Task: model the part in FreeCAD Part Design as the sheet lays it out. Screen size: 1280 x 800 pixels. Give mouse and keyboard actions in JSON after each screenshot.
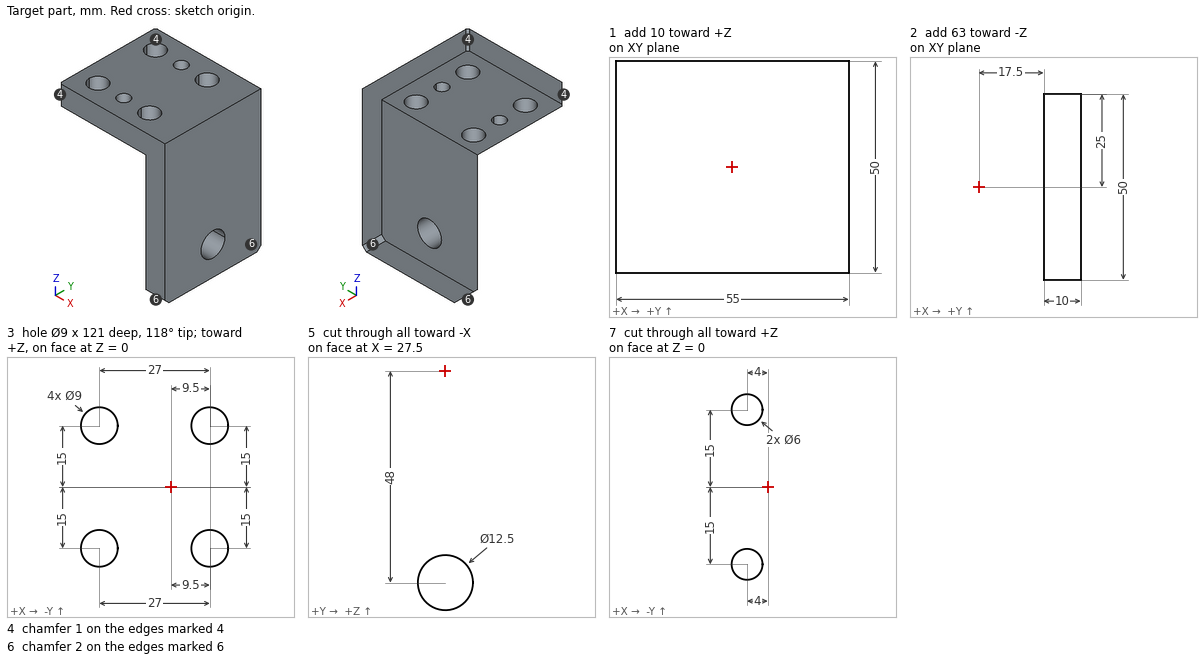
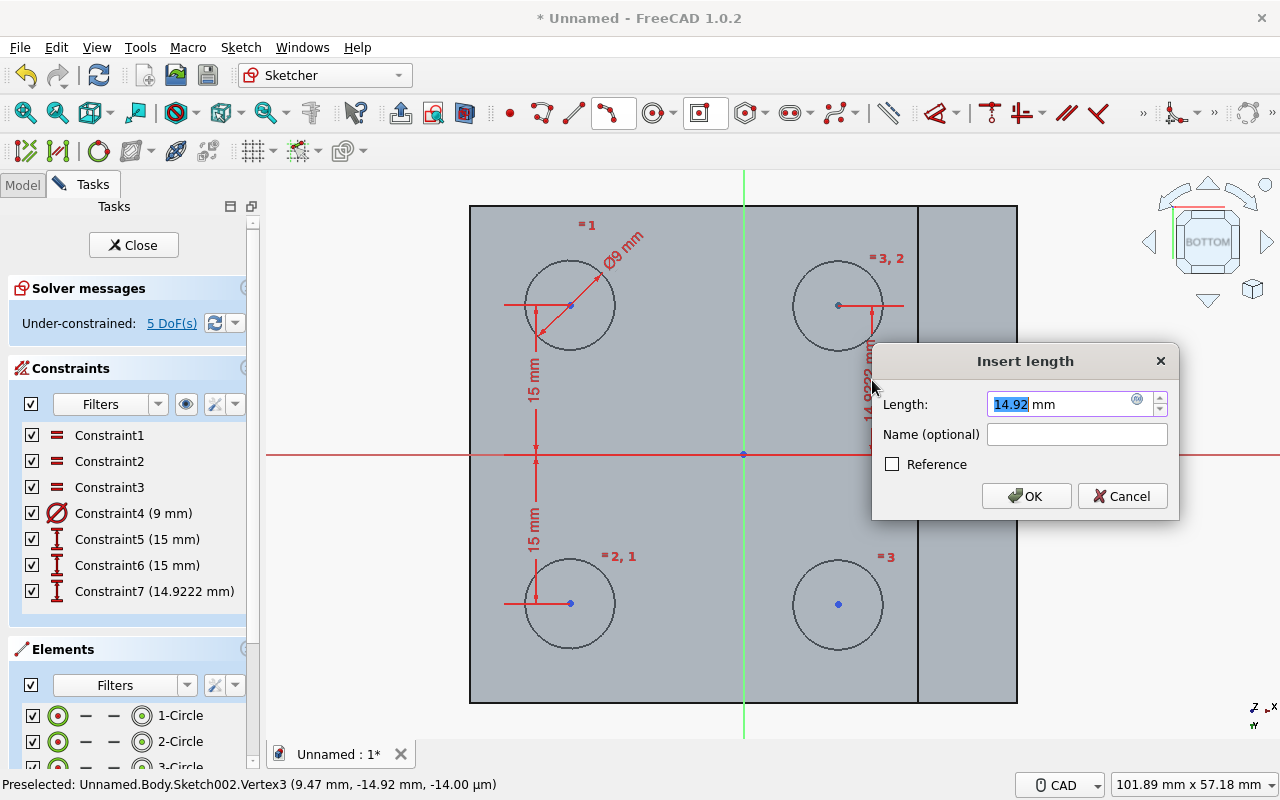
{"action": "type", "text": "15"}
{"action": "key", "text": "Return"}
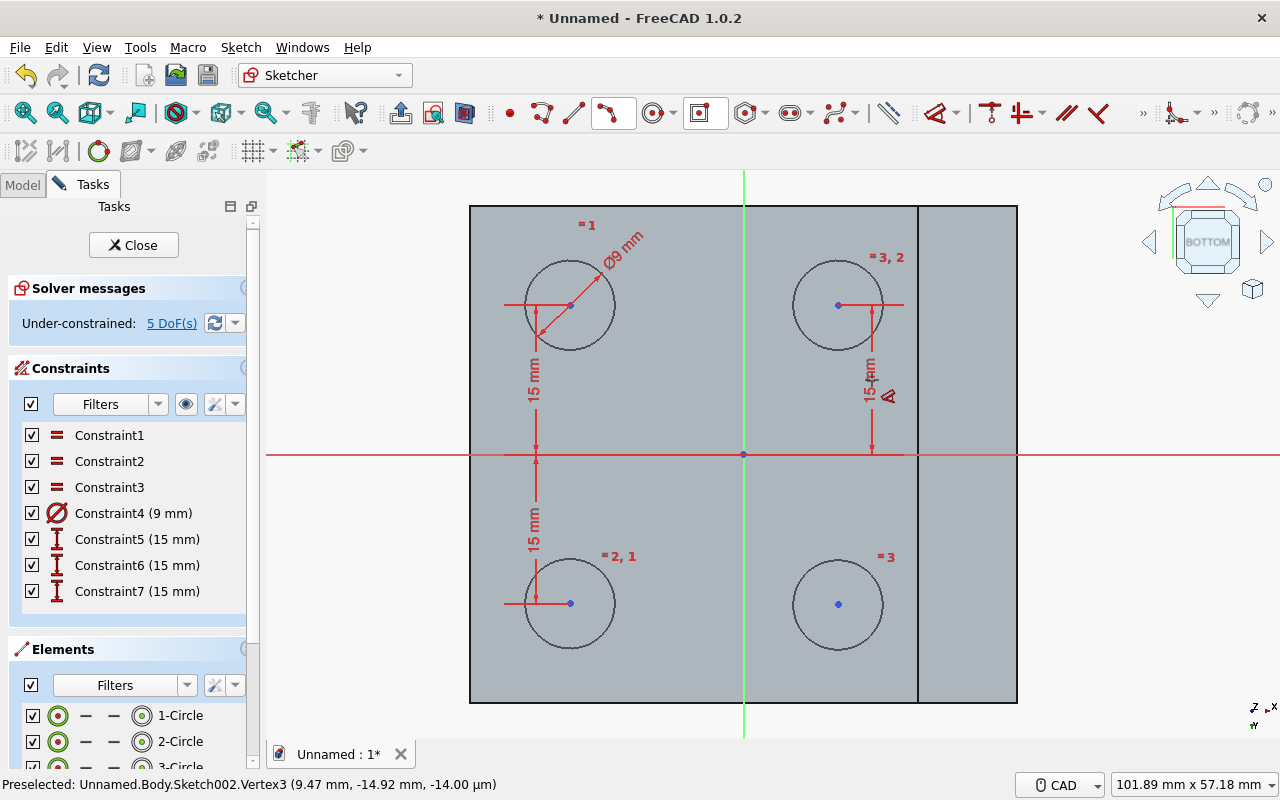
{"action": "left_click", "coordinate": [838, 605]}
{"action": "left_click", "coordinate": [872, 530]}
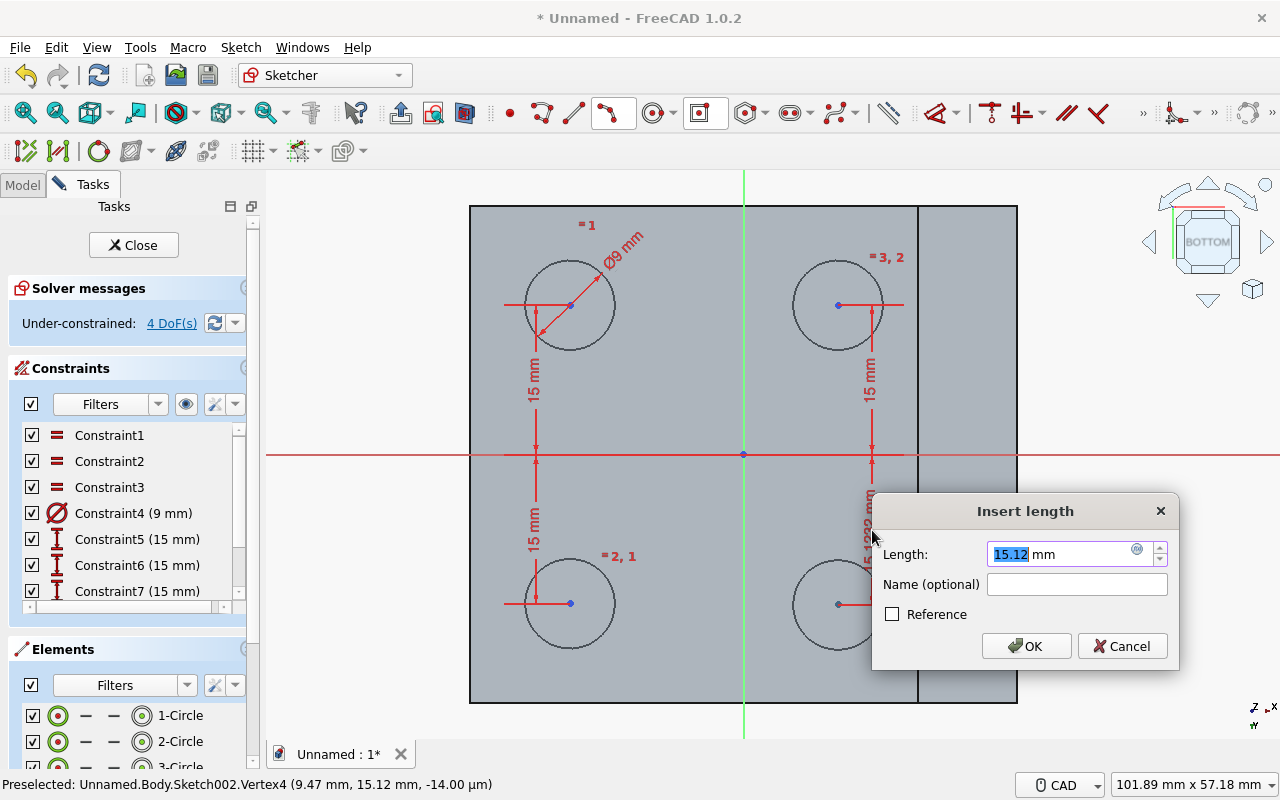
{"action": "type", "text": "15"}
{"action": "key", "text": "Return"}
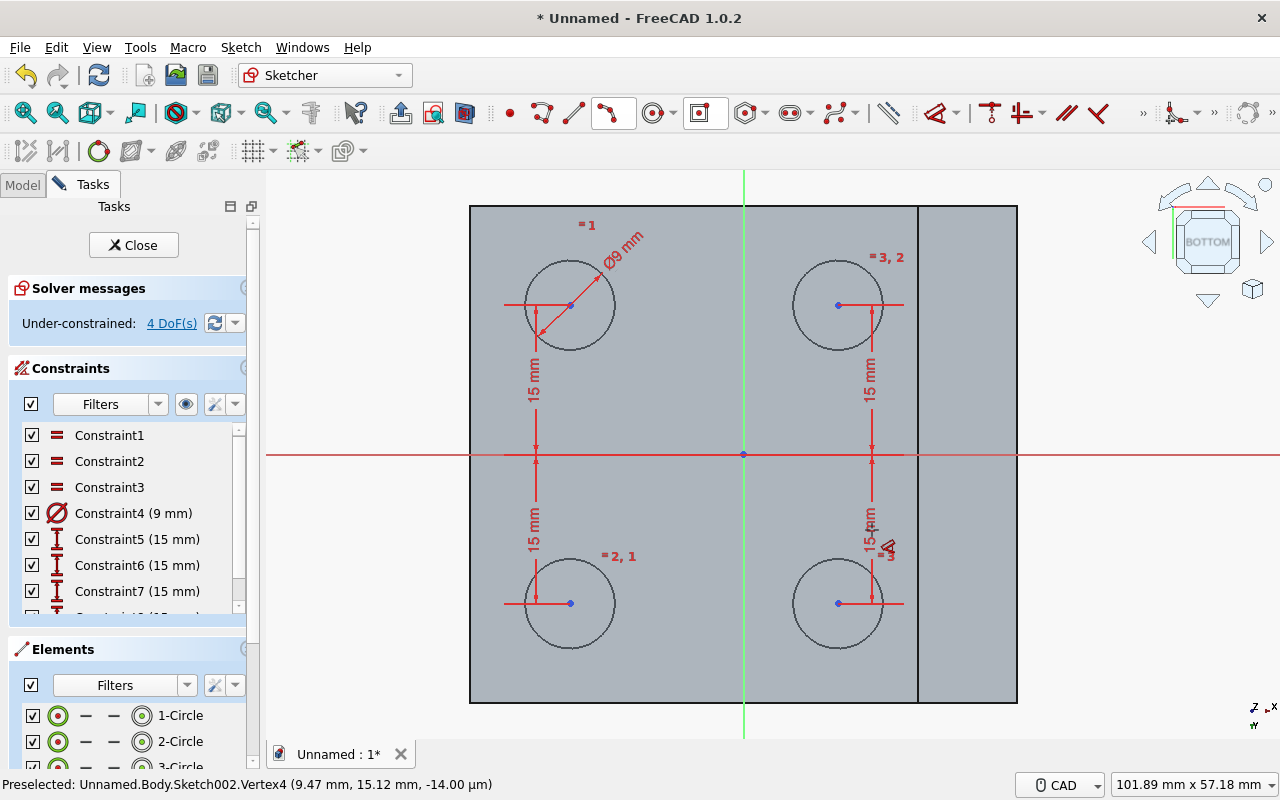
{"action": "left_click", "coordinate": [838, 305]}
{"action": "left_click", "coordinate": [791, 271]}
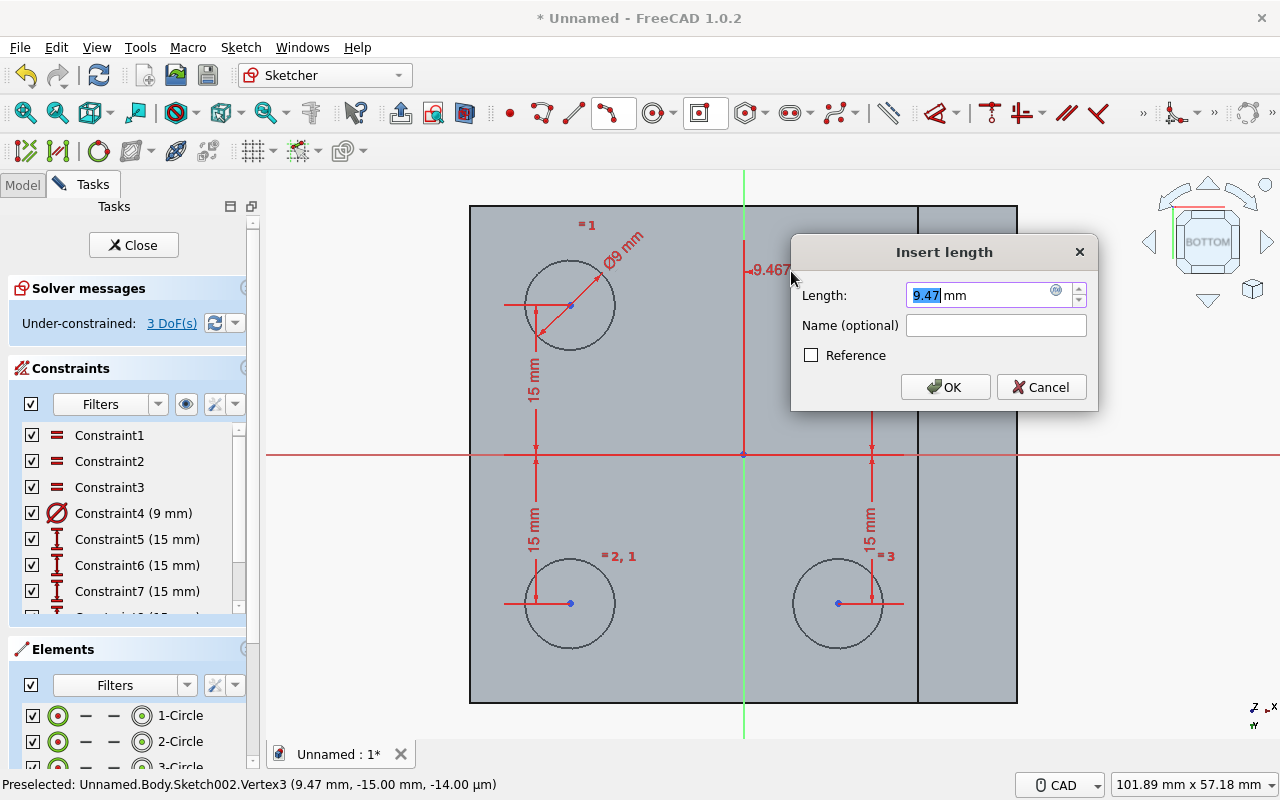
{"action": "type", "text": "9.5"}
{"action": "key", "text": "Return"}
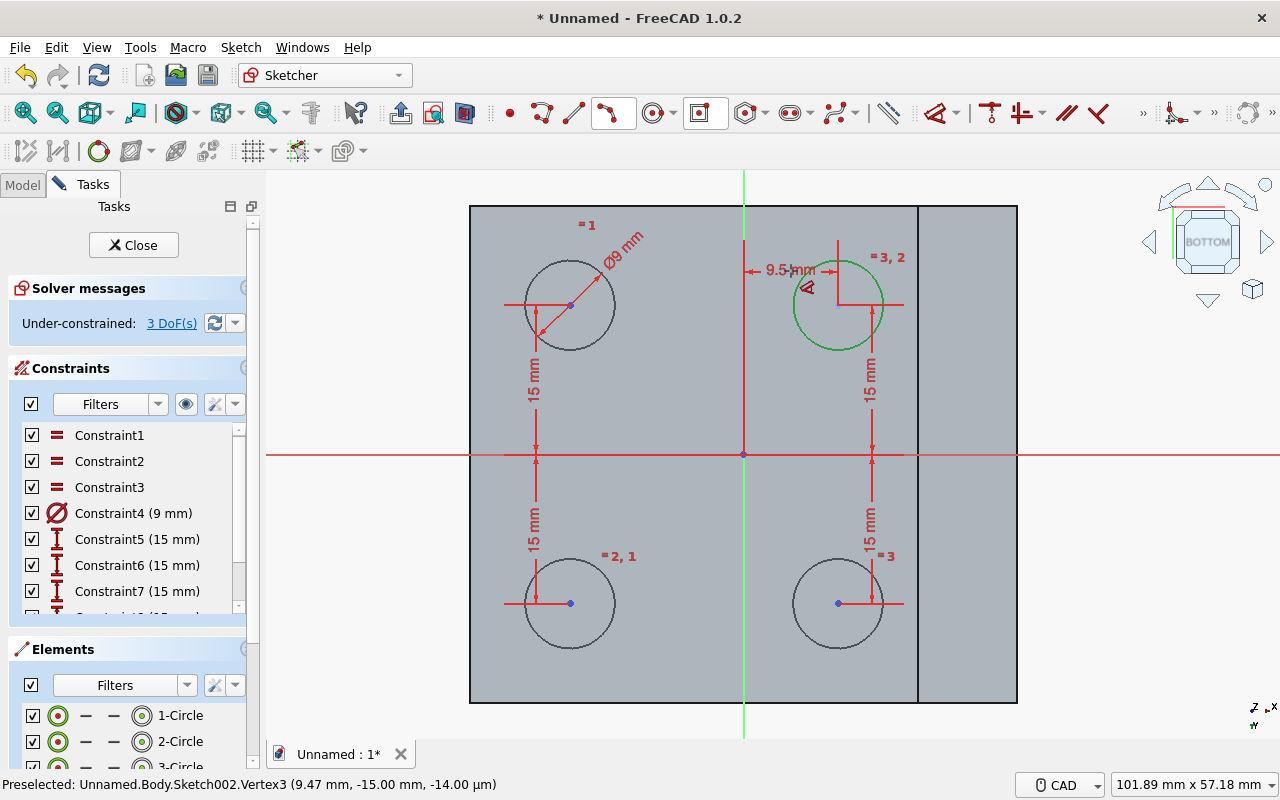
{"action": "left_click", "coordinate": [838, 604]}
{"action": "left_click", "coordinate": [791, 638]}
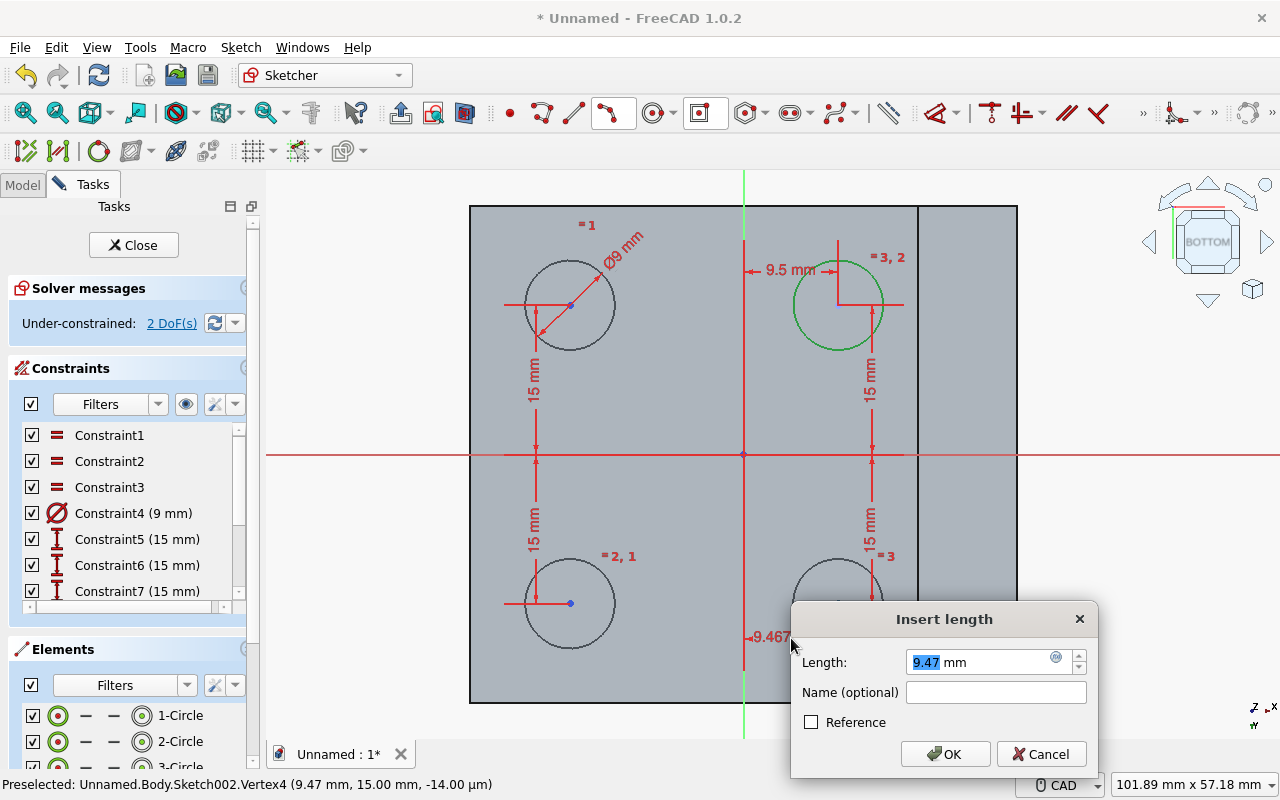
{"action": "type", "text": "9.5"}
{"action": "key", "text": "Return"}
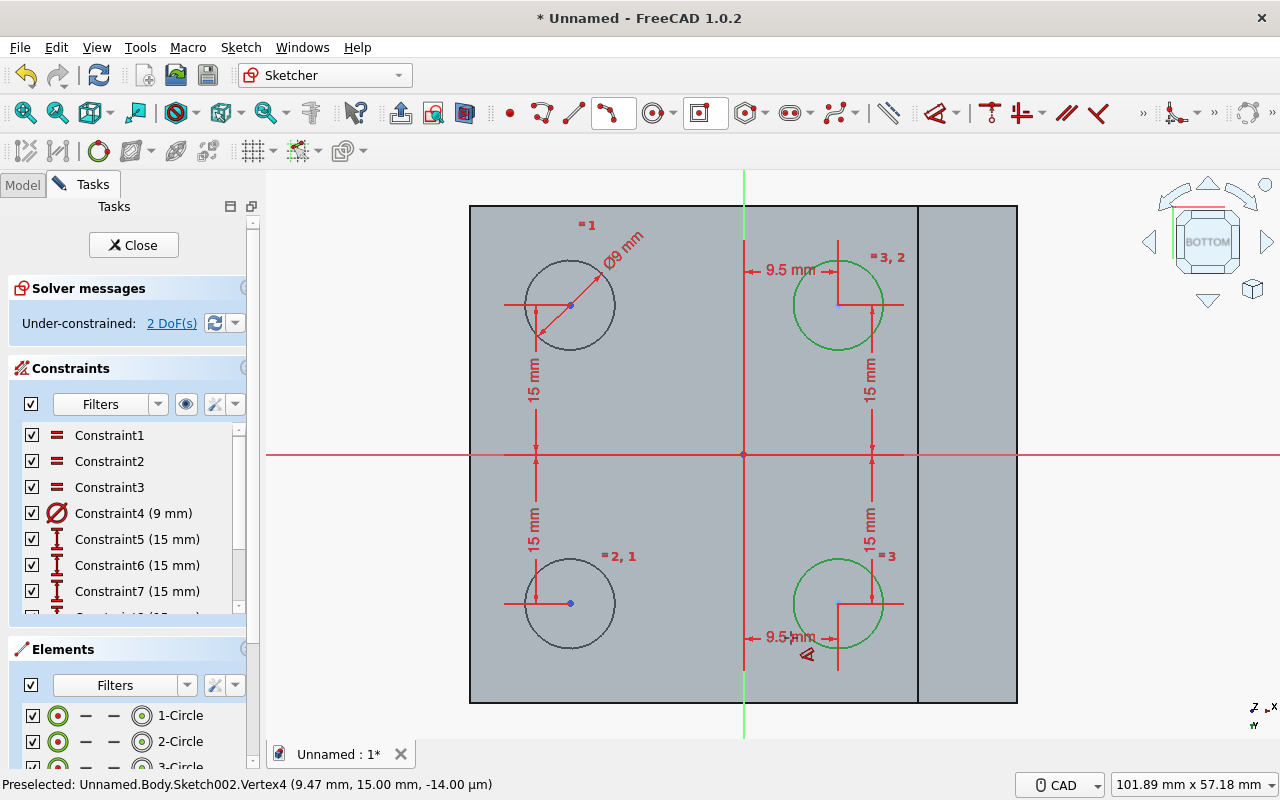
{"action": "left_click", "coordinate": [570, 305]}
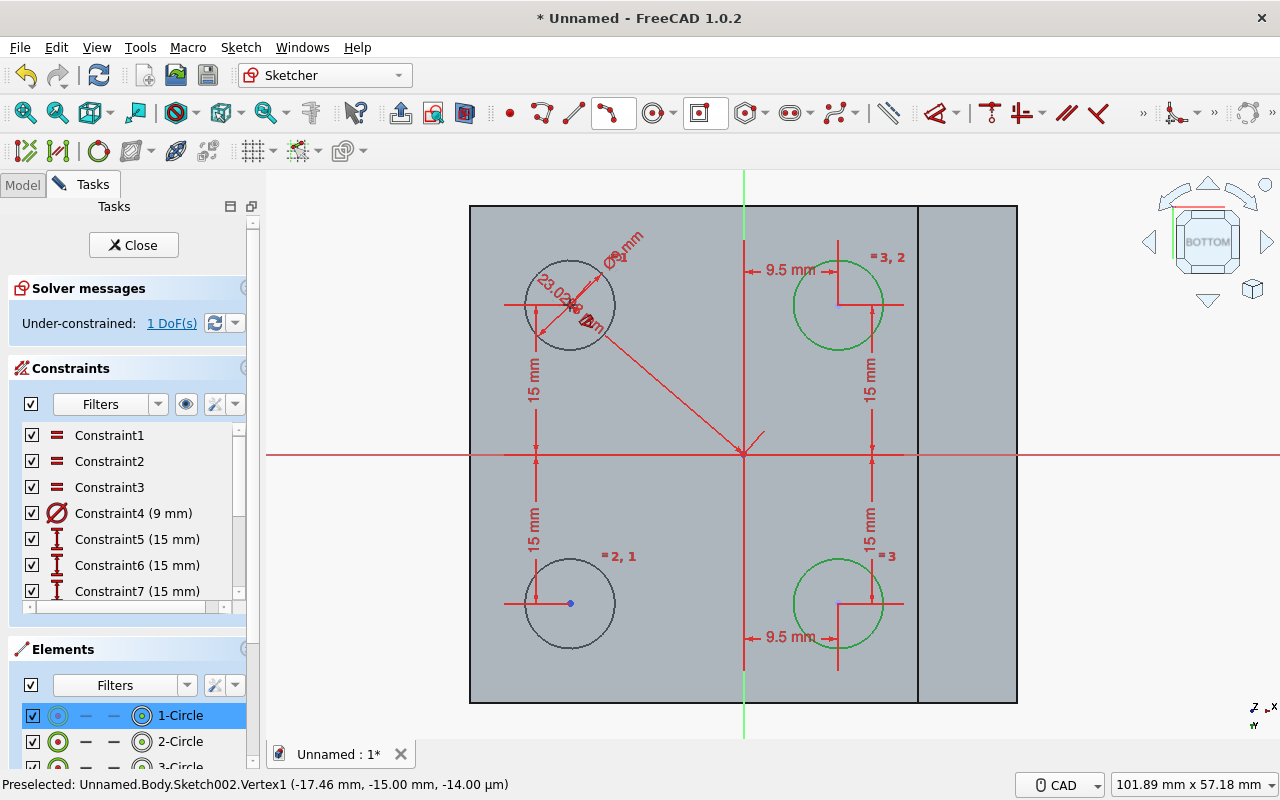
{"action": "left_click", "coordinate": [838, 305]}
{"action": "left_click", "coordinate": [704, 271]}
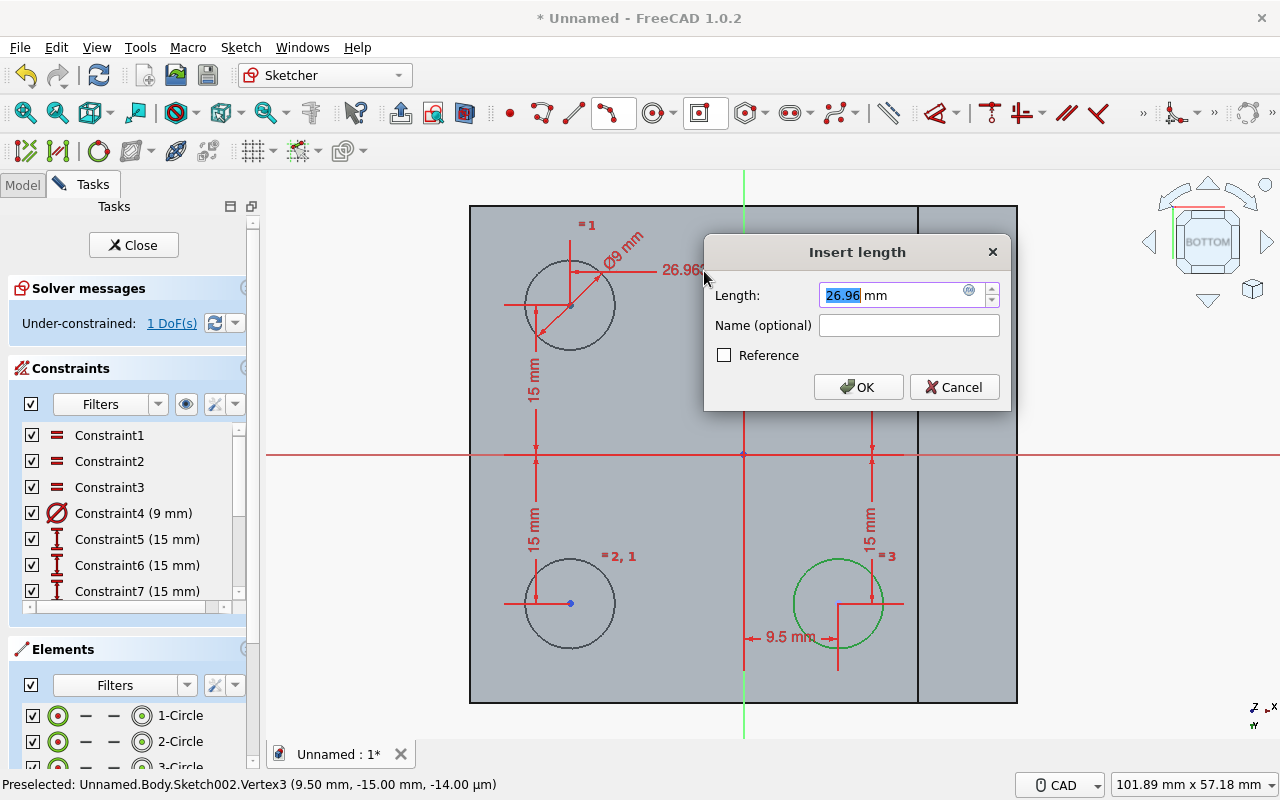
{"action": "type", "text": "27"}
{"action": "key", "text": "Return"}